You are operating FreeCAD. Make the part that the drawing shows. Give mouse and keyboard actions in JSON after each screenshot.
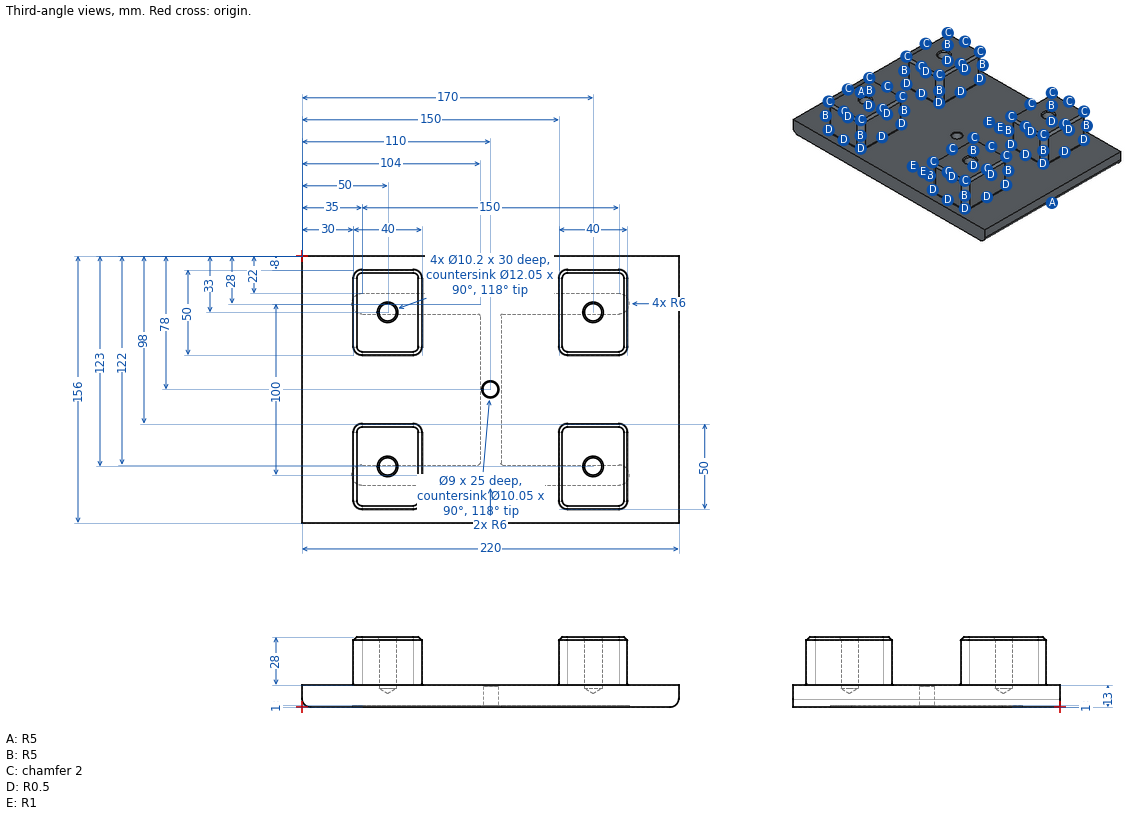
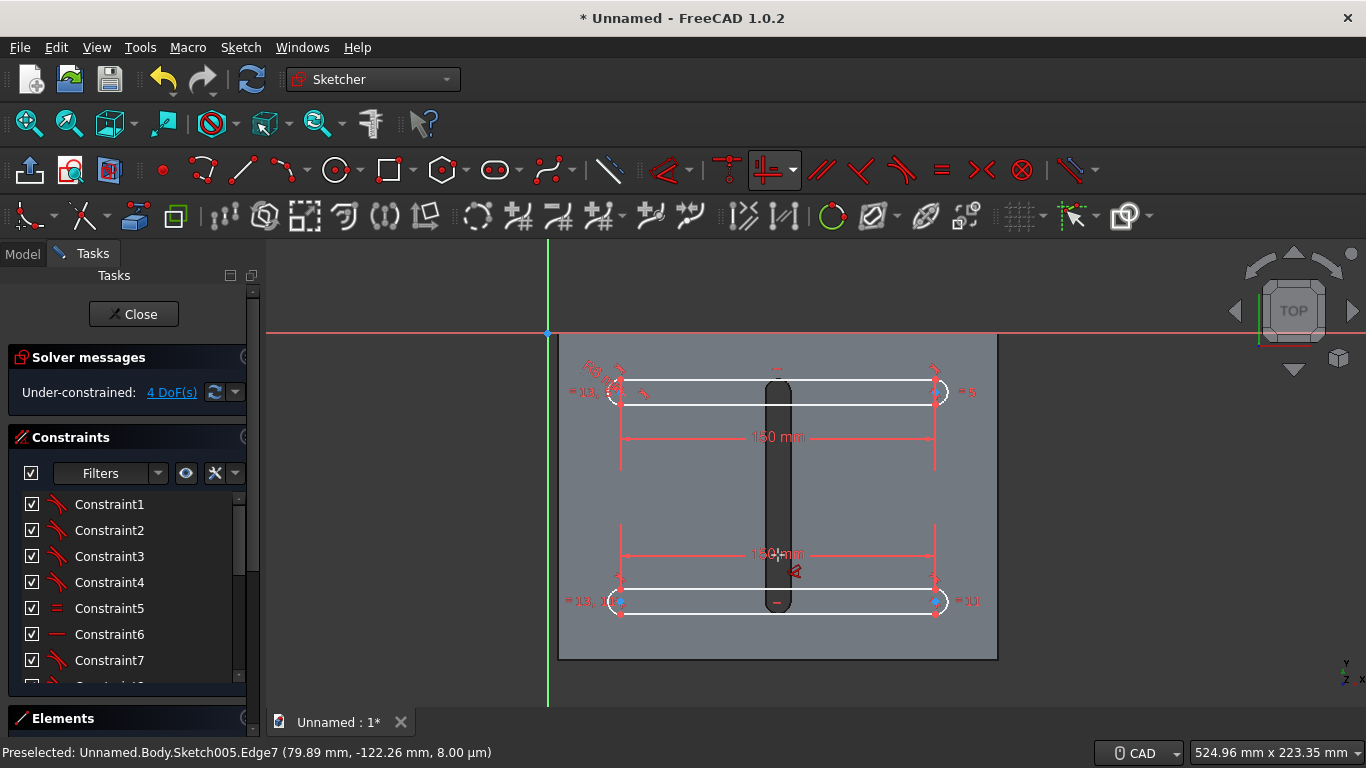
{"action": "left_click", "coordinate": [621, 380]}
{"action": "left_click", "coordinate": [584, 299]}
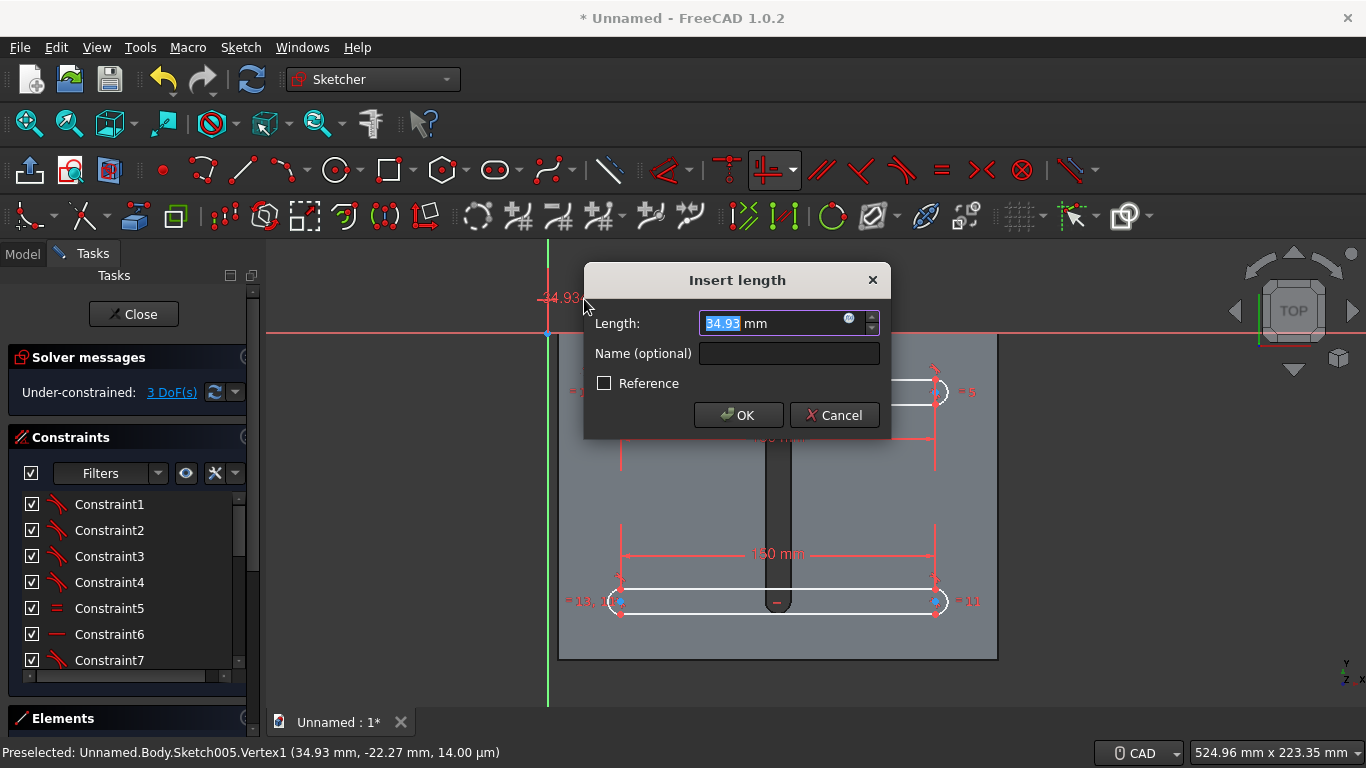
{"action": "type", "text": "35"}
{"action": "key", "text": "Return"}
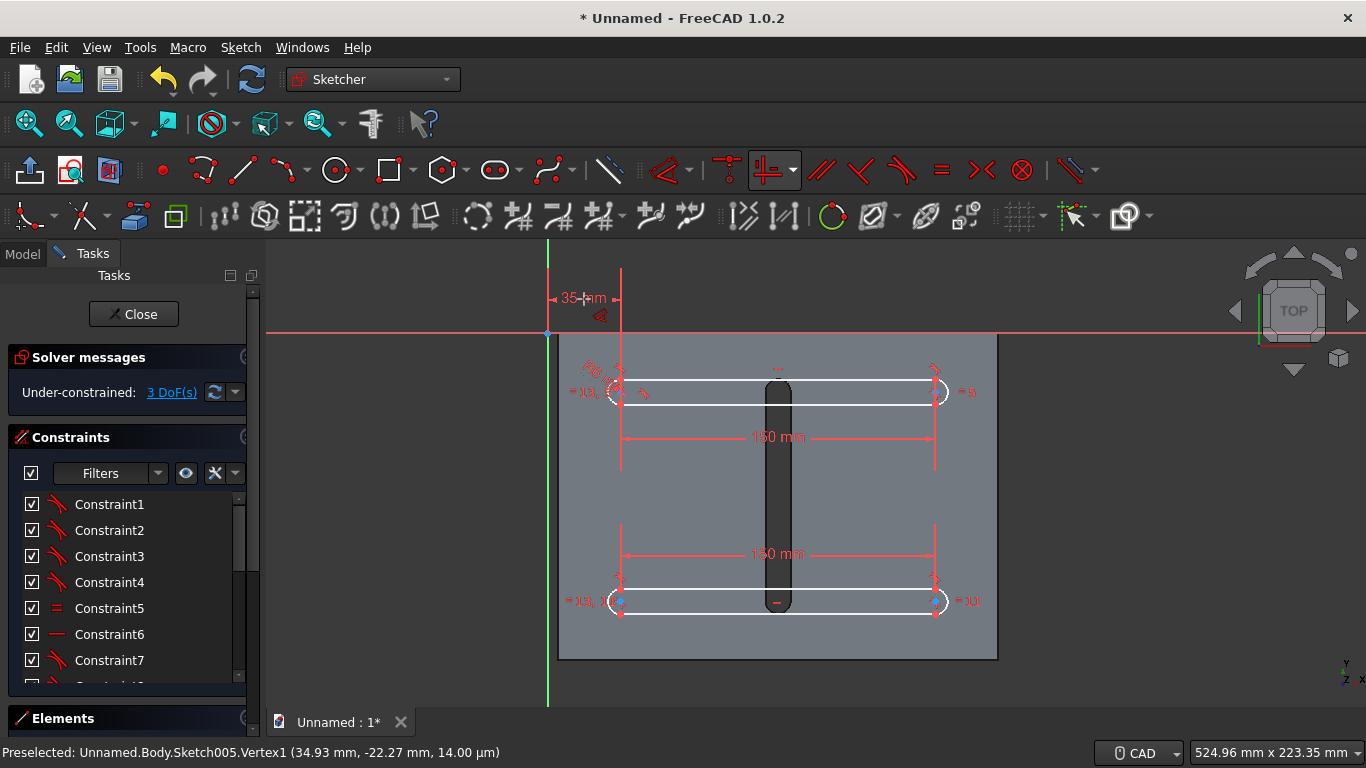
{"action": "left_click", "coordinate": [621, 380]}
{"action": "left_click", "coordinate": [514, 356]}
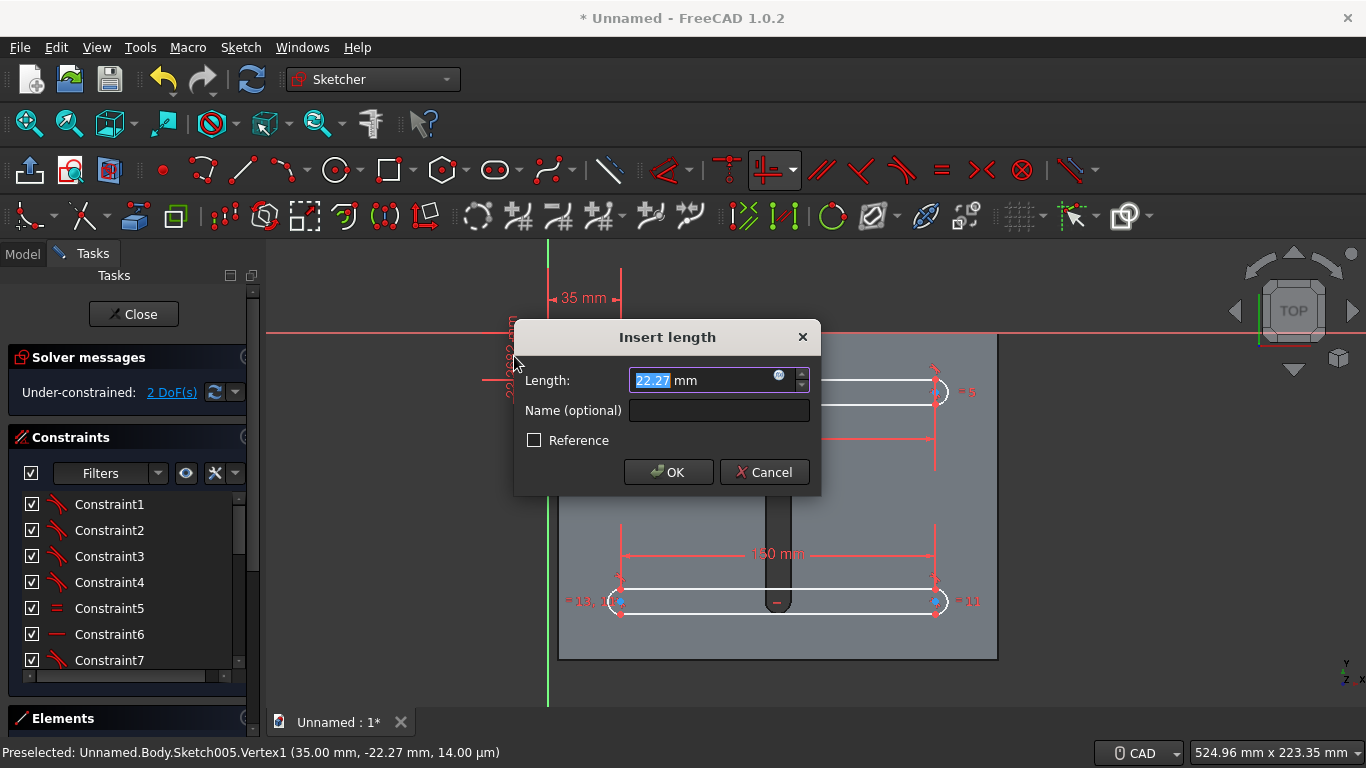
{"action": "type", "text": "22"}
{"action": "key", "text": "Return"}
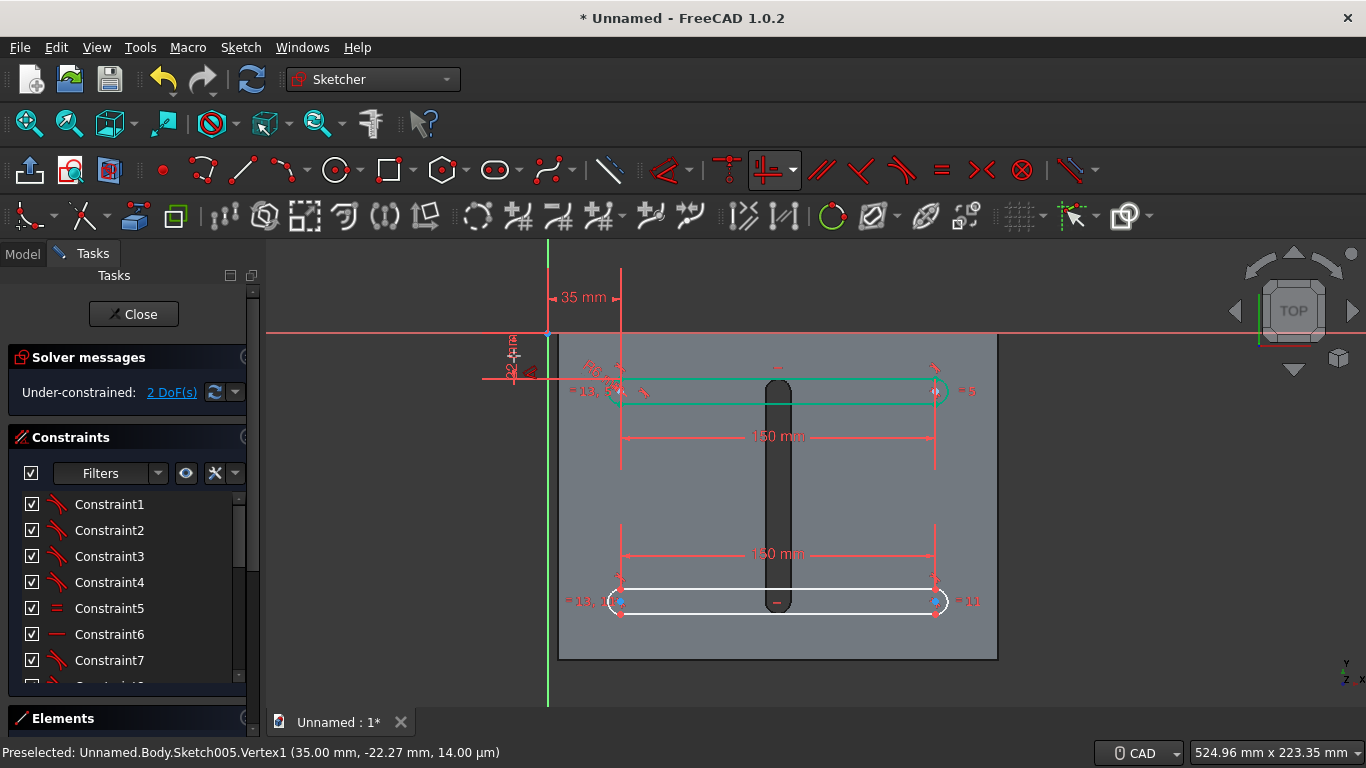
{"action": "left_click", "coordinate": [621, 589]}
{"action": "left_click", "coordinate": [584, 623]}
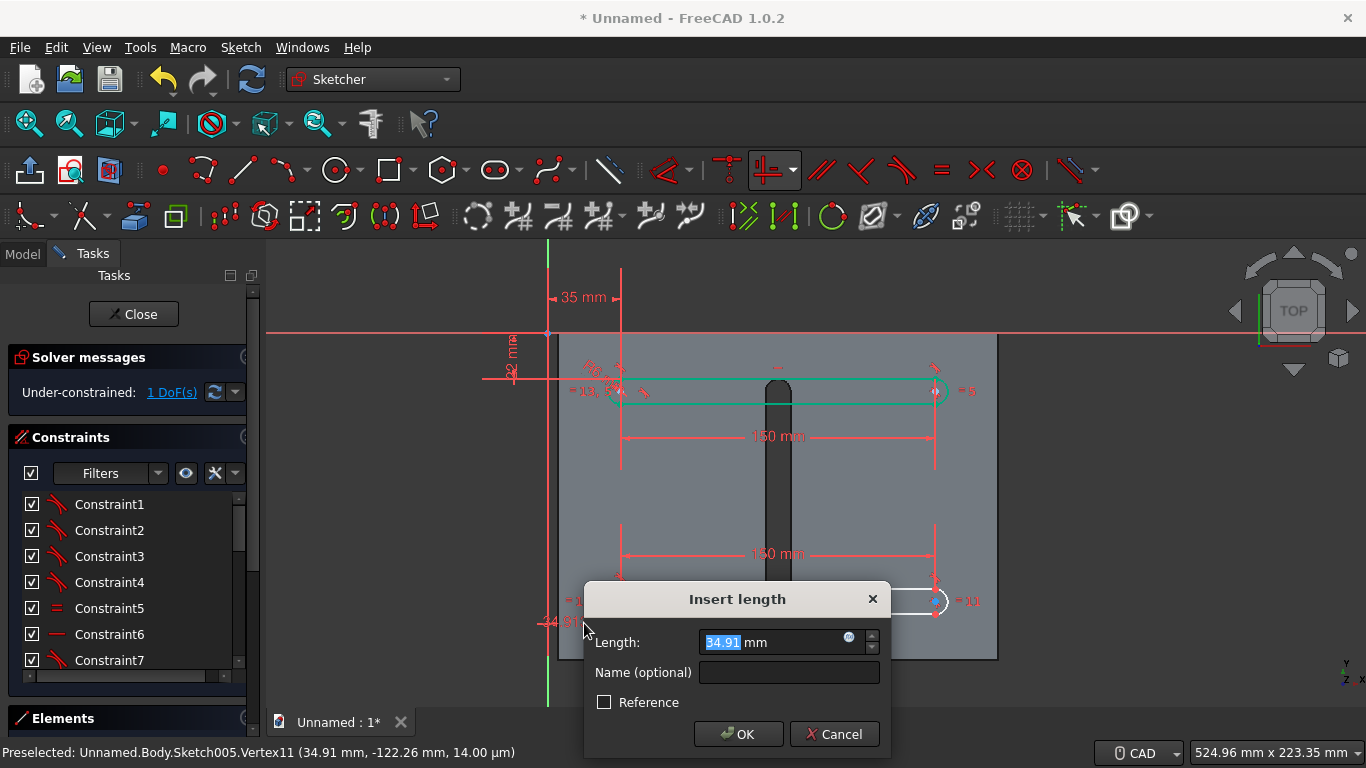
{"action": "type", "text": "35"}
{"action": "key", "text": "Return"}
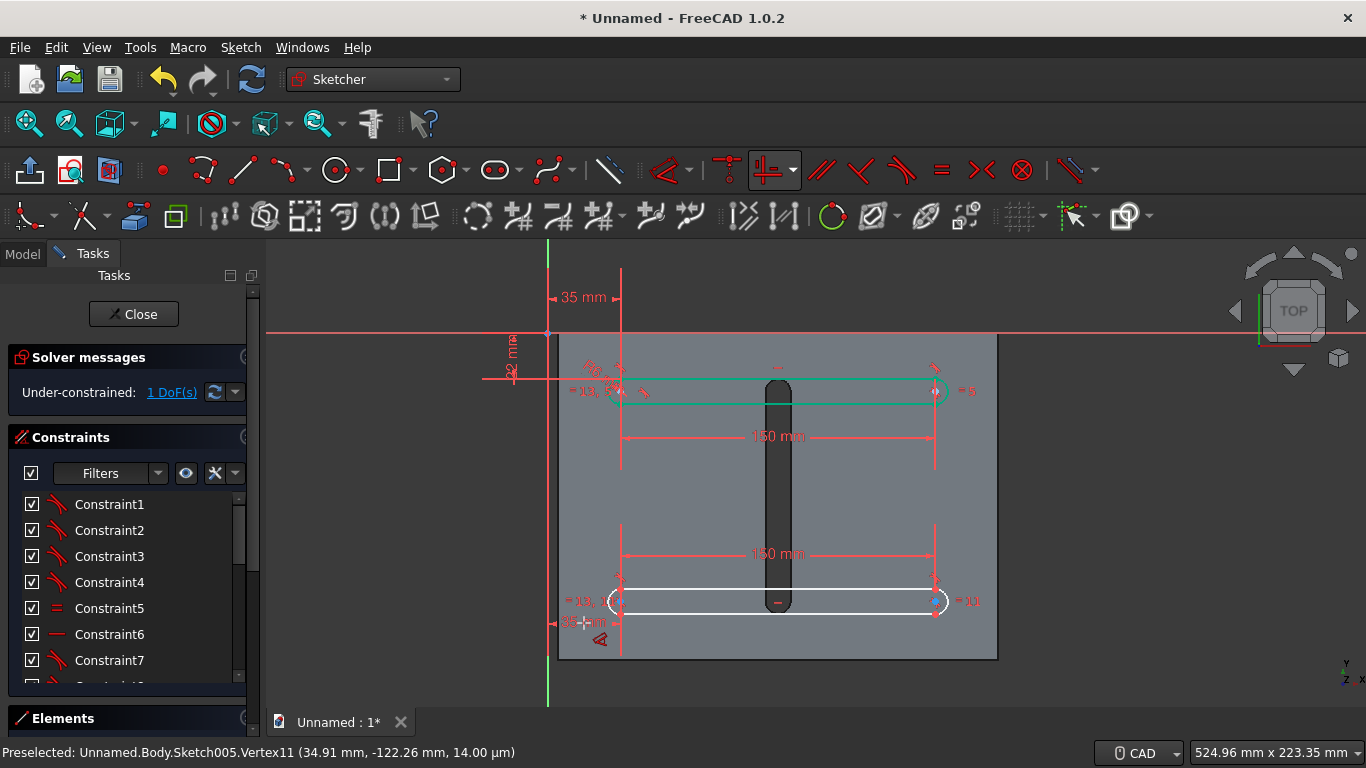
{"action": "left_click", "coordinate": [621, 589]}
{"action": "left_click", "coordinate": [514, 461]}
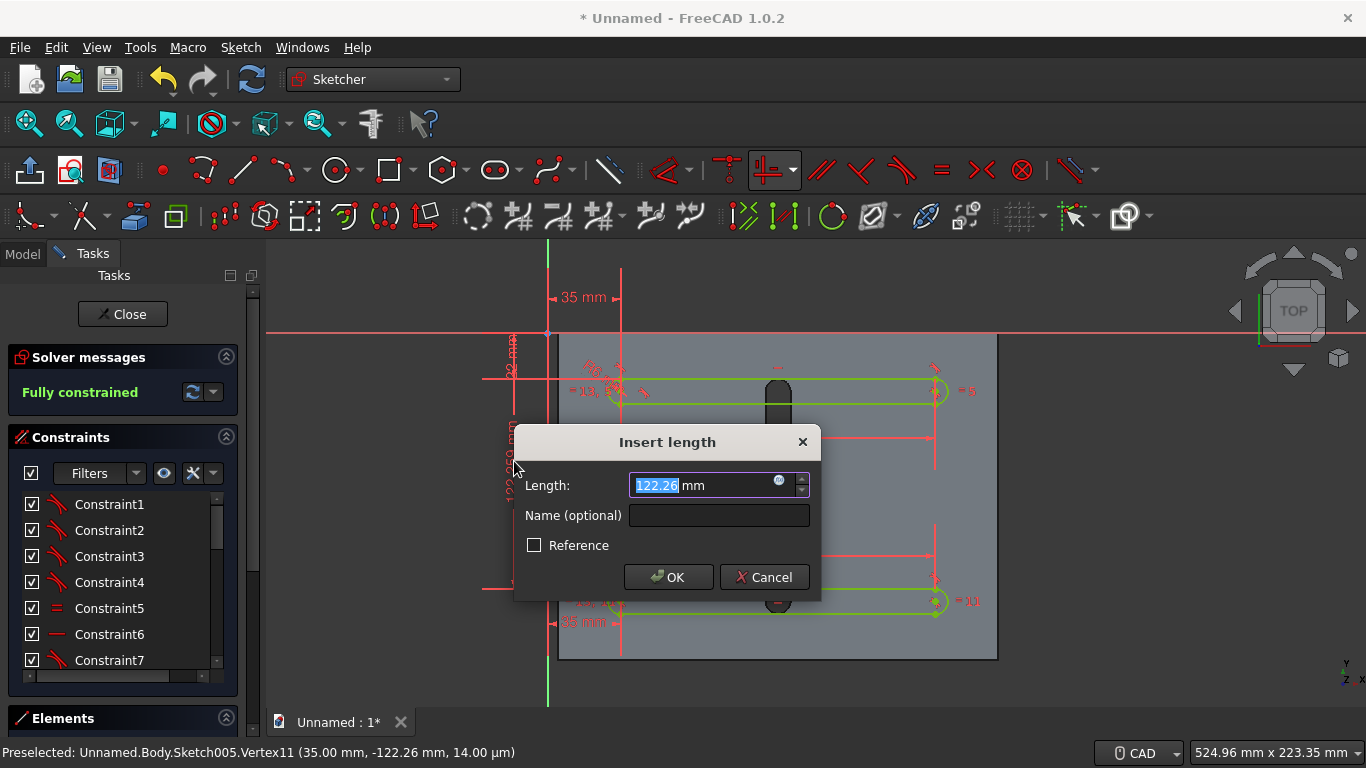
{"action": "type", "text": "122"}
{"action": "key", "text": "Return"}
{"action": "key", "text": "Escape"}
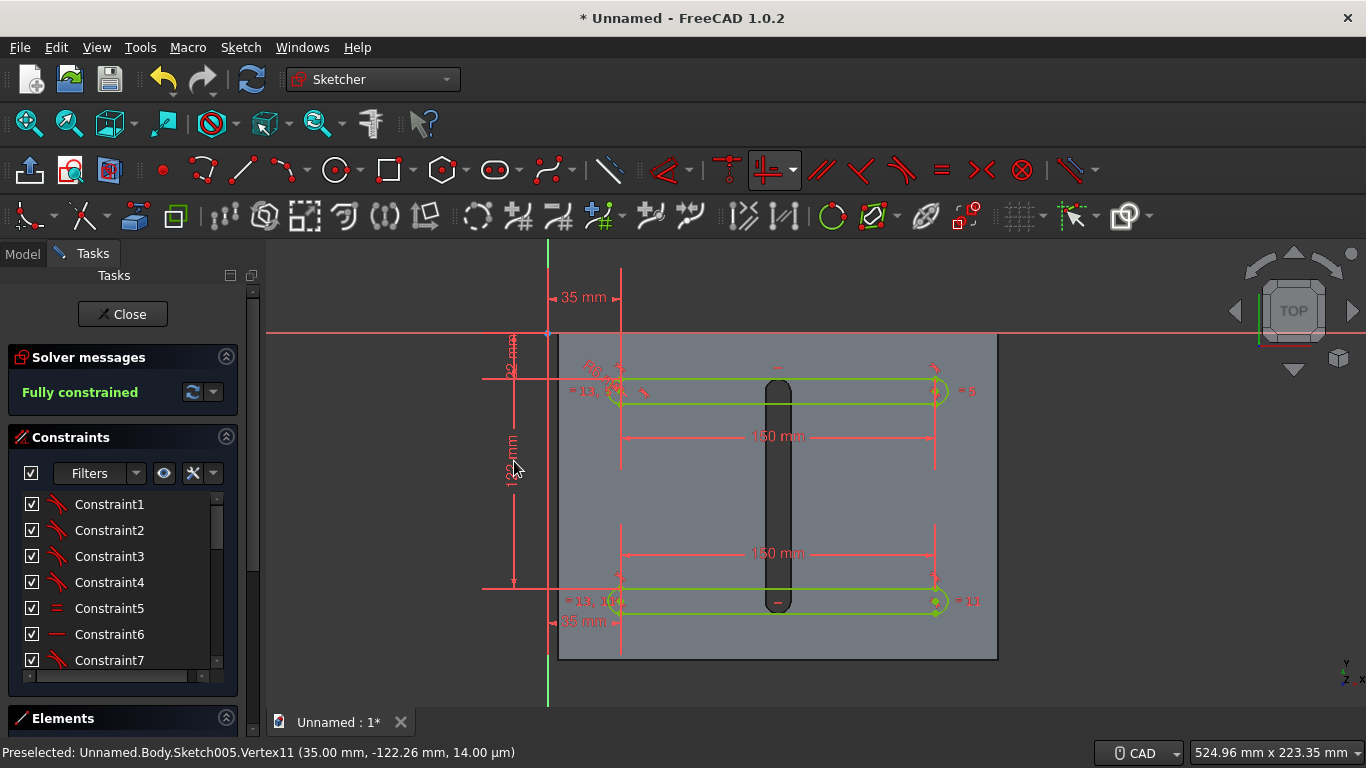
{"action": "left_click", "coordinate": [123, 314]}